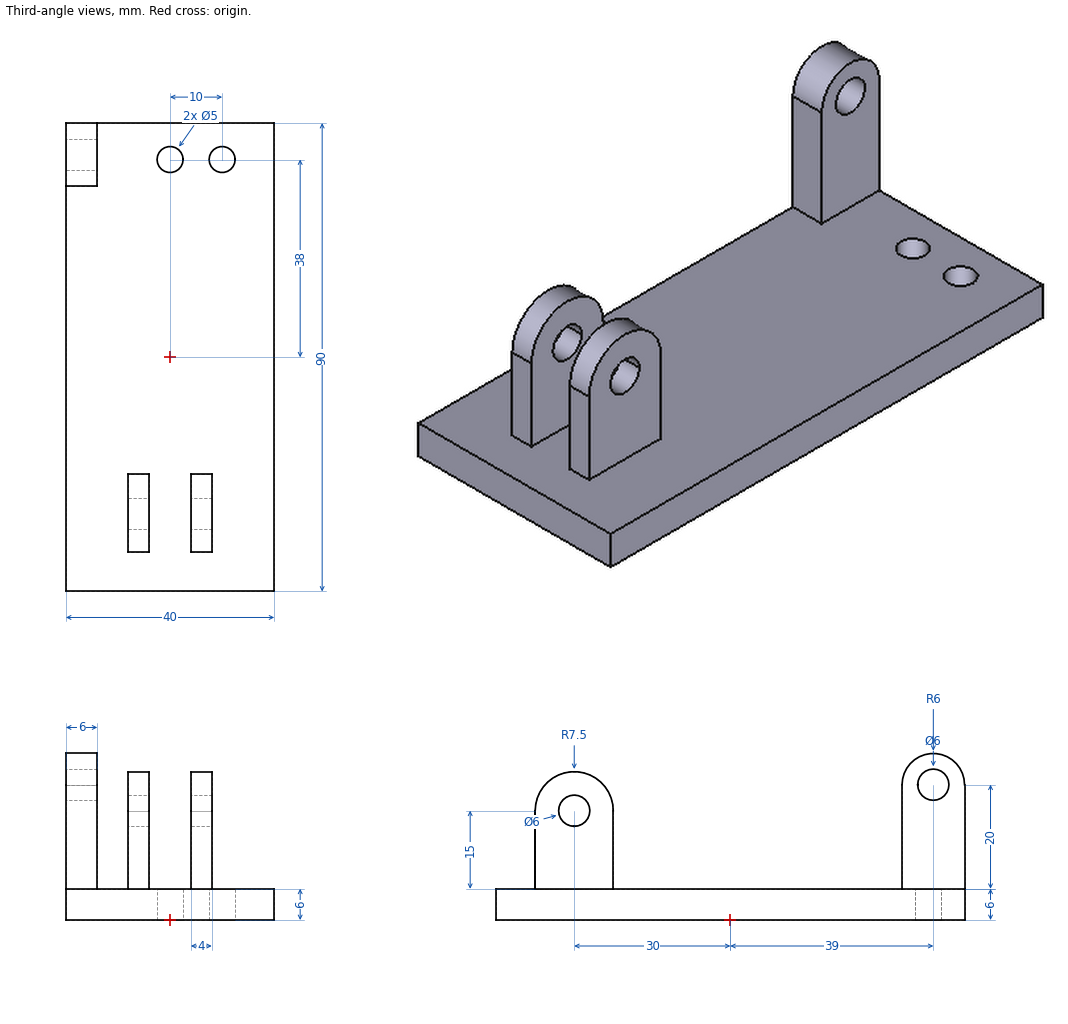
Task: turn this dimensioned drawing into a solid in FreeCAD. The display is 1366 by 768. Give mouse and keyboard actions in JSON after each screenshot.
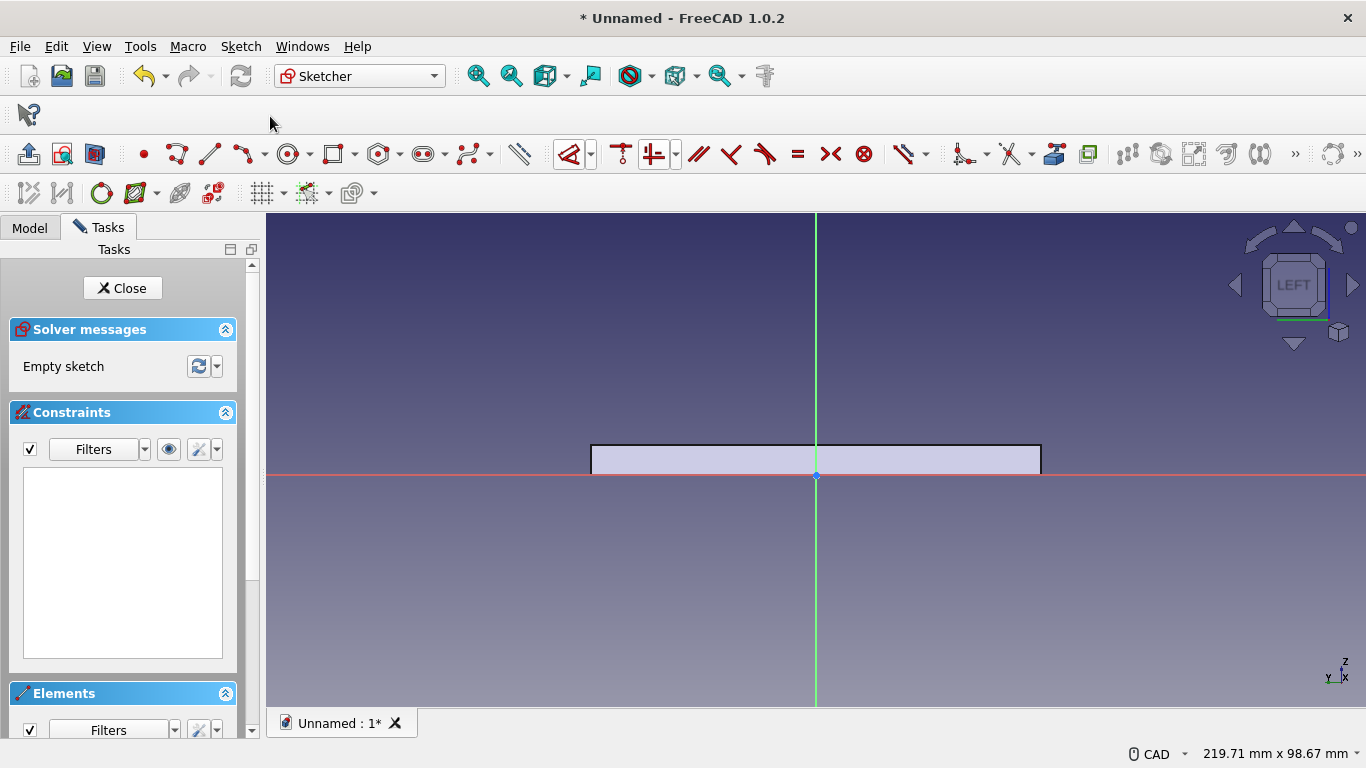
{"action": "scroll", "coordinate": [650, 316], "scroll_direction": "up", "scroll_amount": 3}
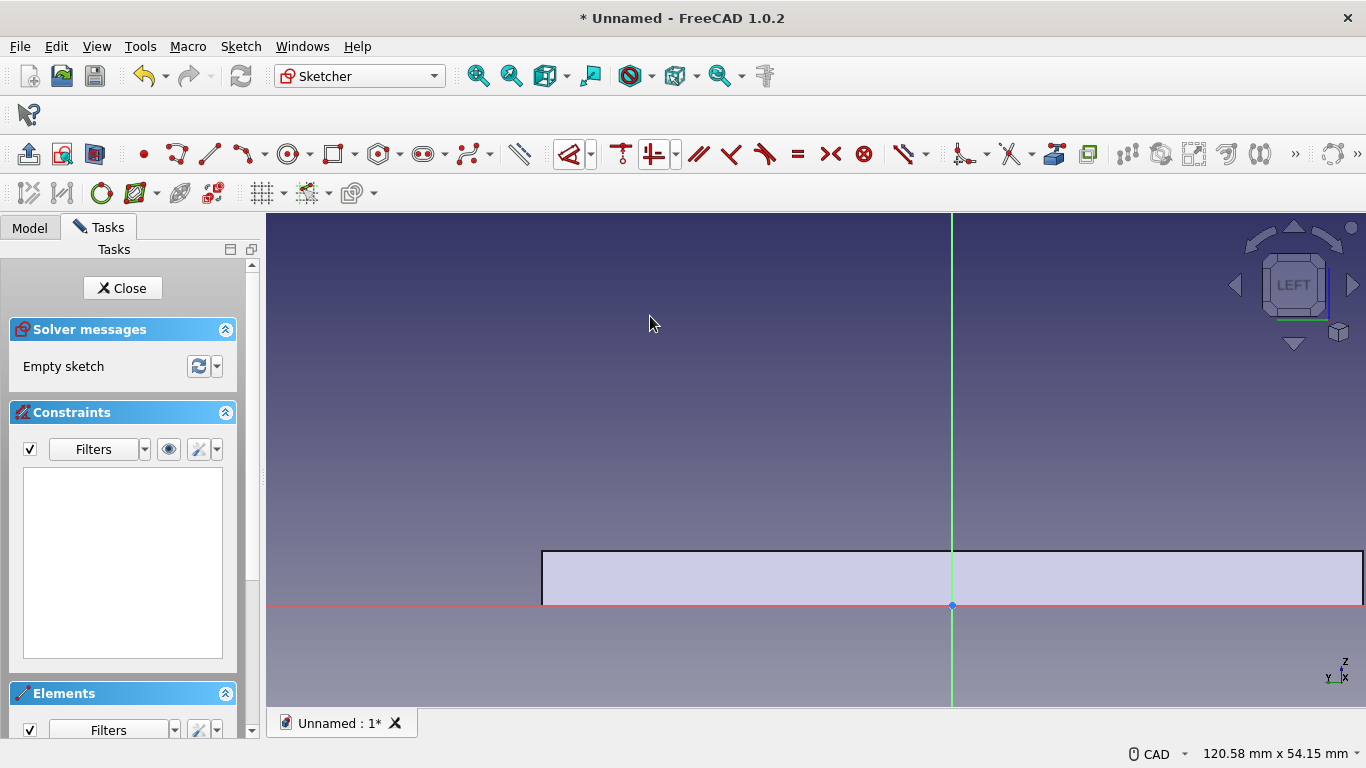
{"action": "key", "text": "g m"}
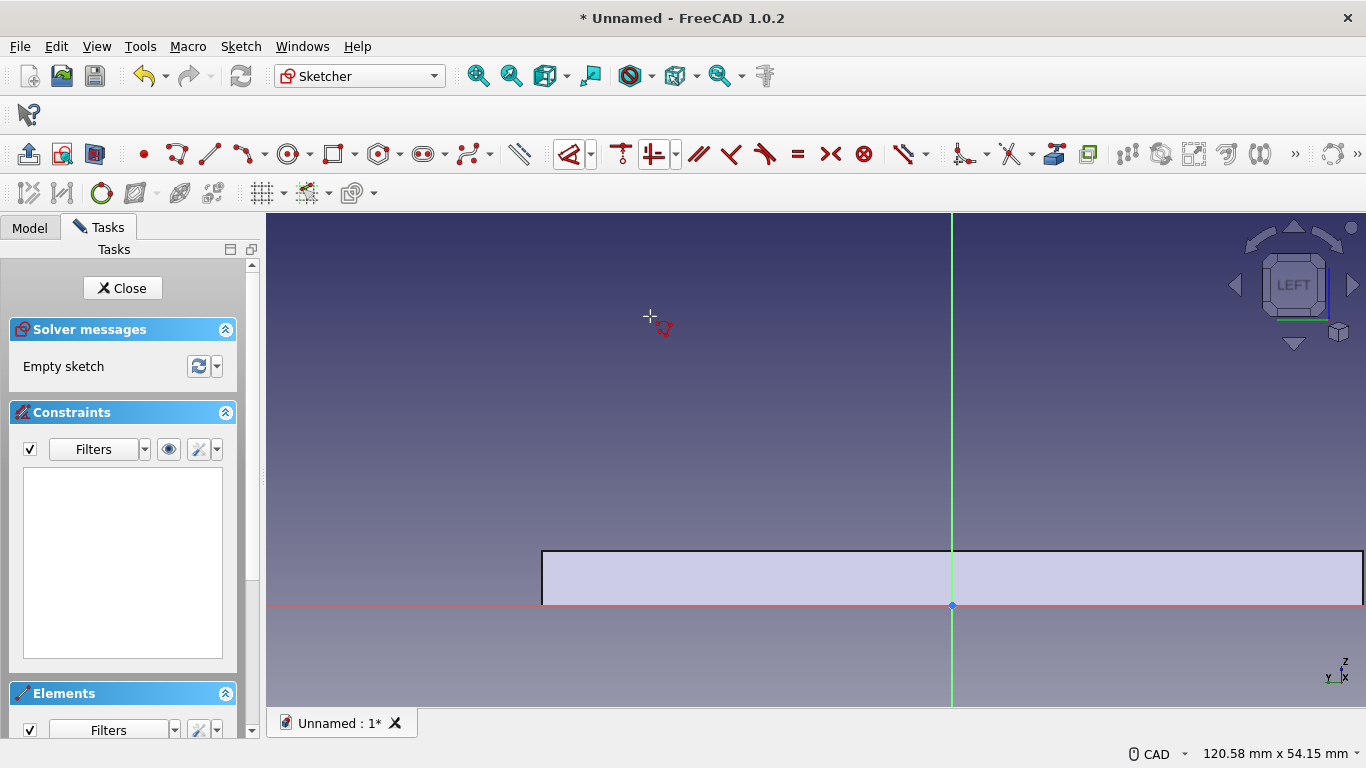
{"action": "left_click", "coordinate": [542, 368]}
{"action": "left_click", "coordinate": [542, 551]}
{"action": "left_click", "coordinate": [651, 551]}
{"action": "left_click", "coordinate": [651, 368]}
{"action": "right_click", "coordinate": [651, 368]}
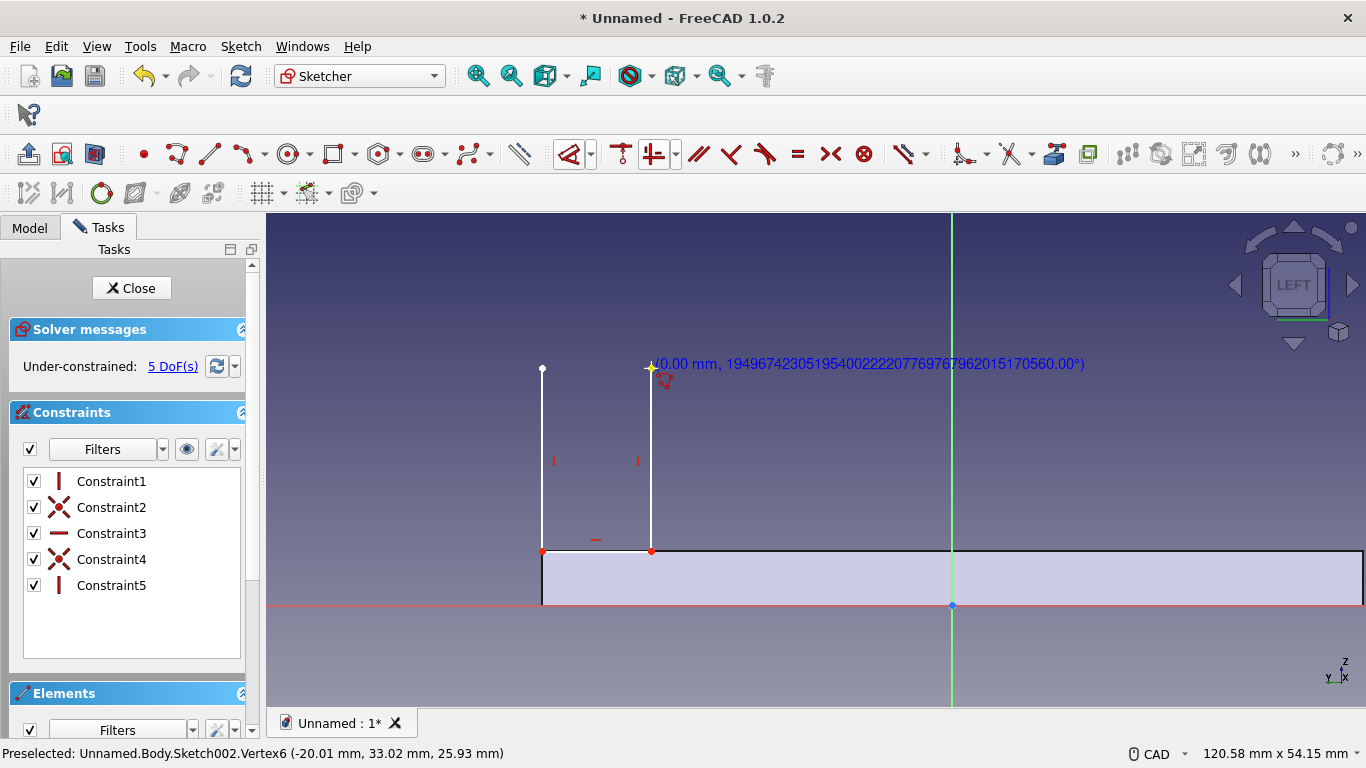
{"action": "key", "text": "g 3 a"}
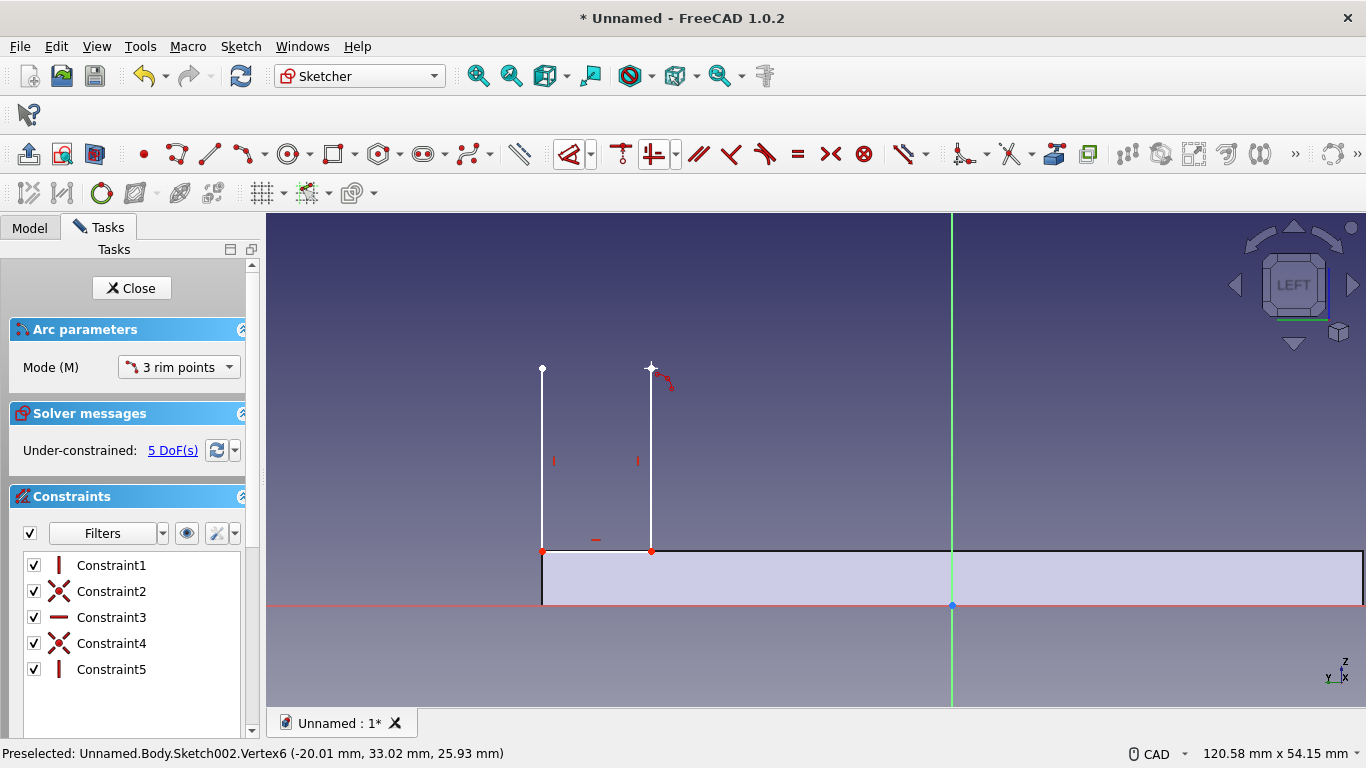
{"action": "left_click", "coordinate": [651, 369]}
{"action": "left_click", "coordinate": [542, 369]}
{"action": "left_click", "coordinate": [596, 314]}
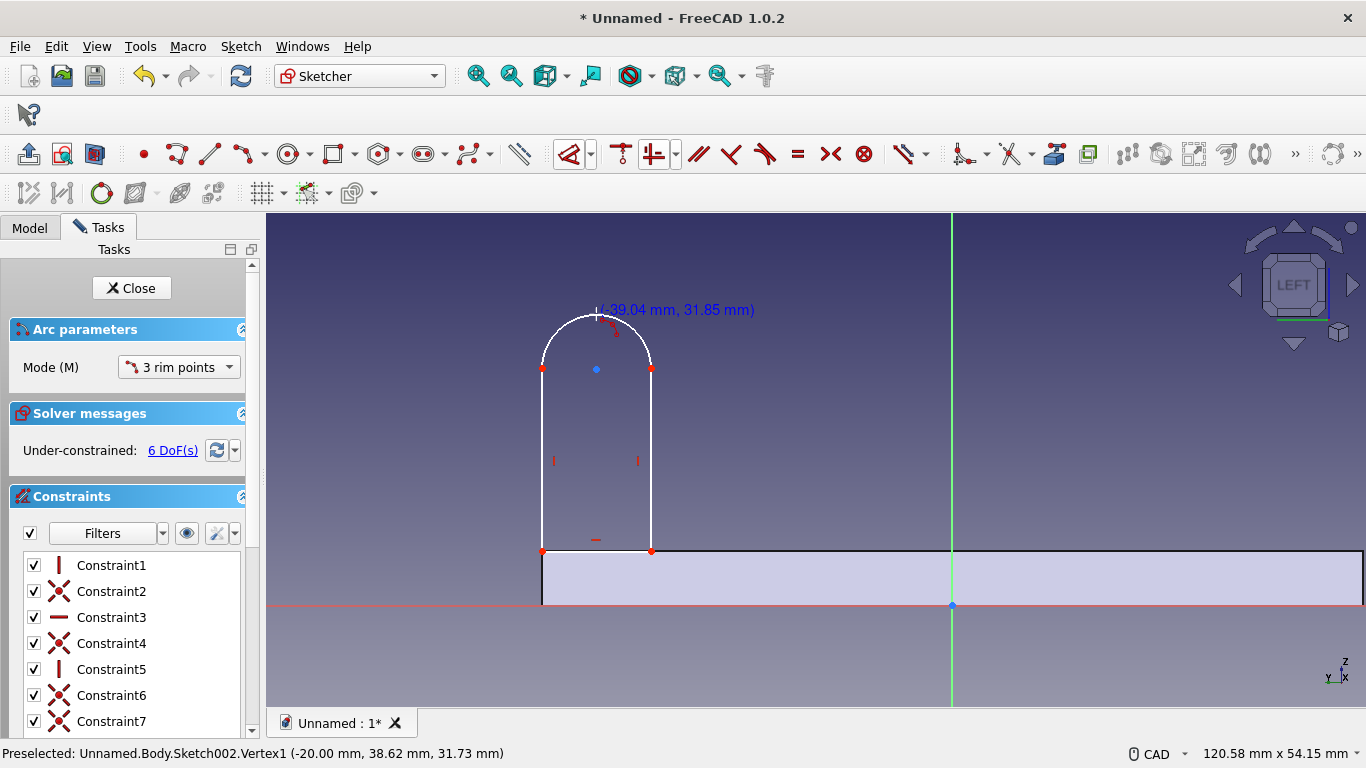
{"action": "key", "text": "g c"}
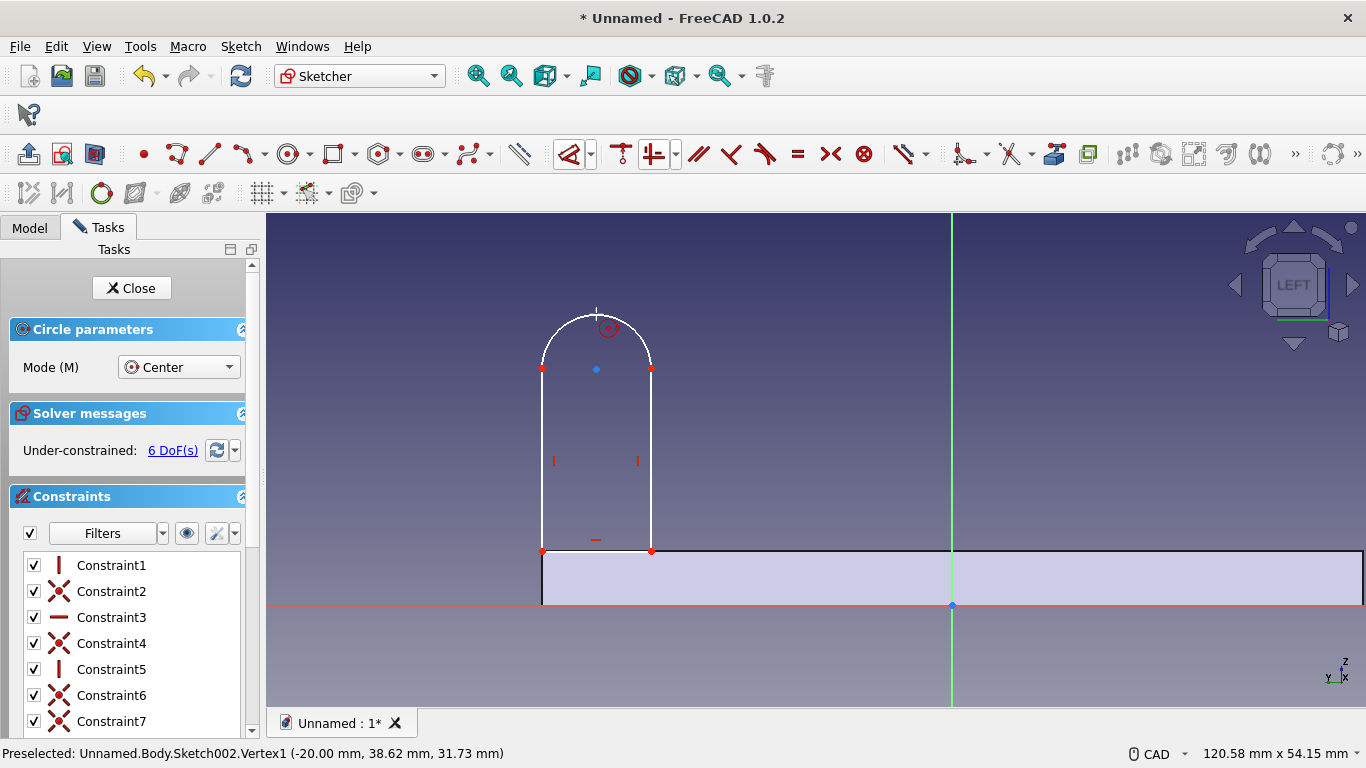
{"action": "left_click", "coordinate": [596, 368]}
{"action": "mouse_move", "coordinate": [616, 349]}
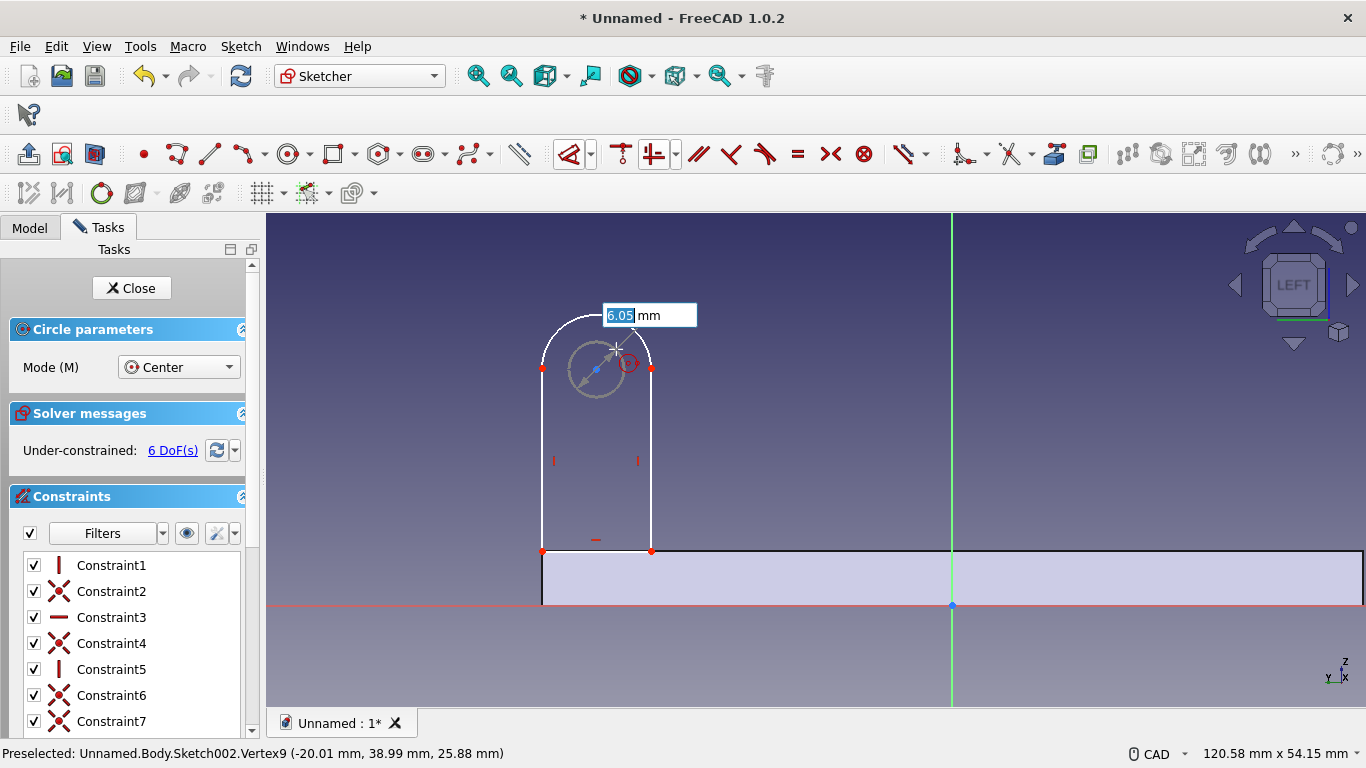
{"action": "type", "text": "6"}
{"action": "key", "text": "Return"}
{"action": "key", "text": "Escape"}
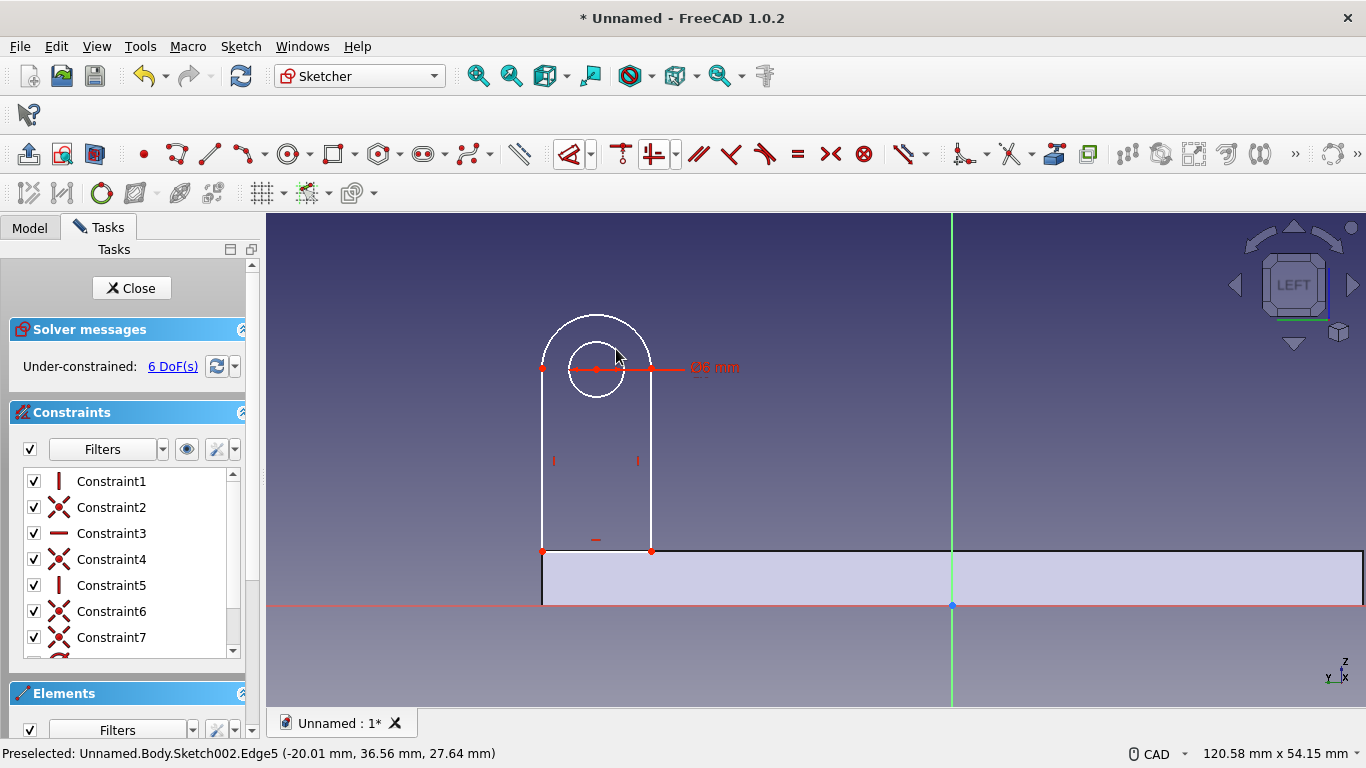
{"action": "left_click", "coordinate": [542, 424]}